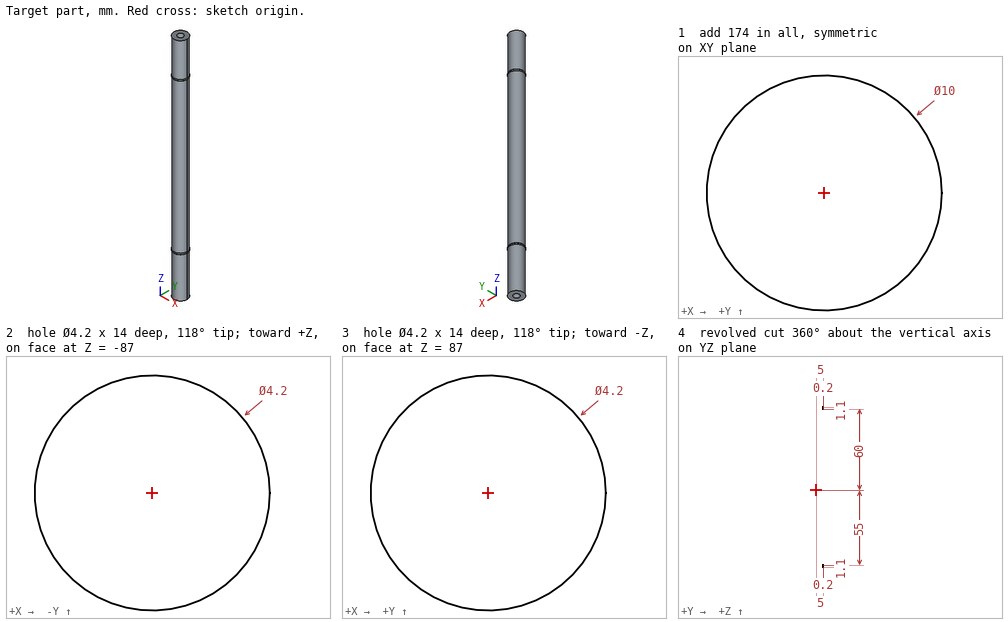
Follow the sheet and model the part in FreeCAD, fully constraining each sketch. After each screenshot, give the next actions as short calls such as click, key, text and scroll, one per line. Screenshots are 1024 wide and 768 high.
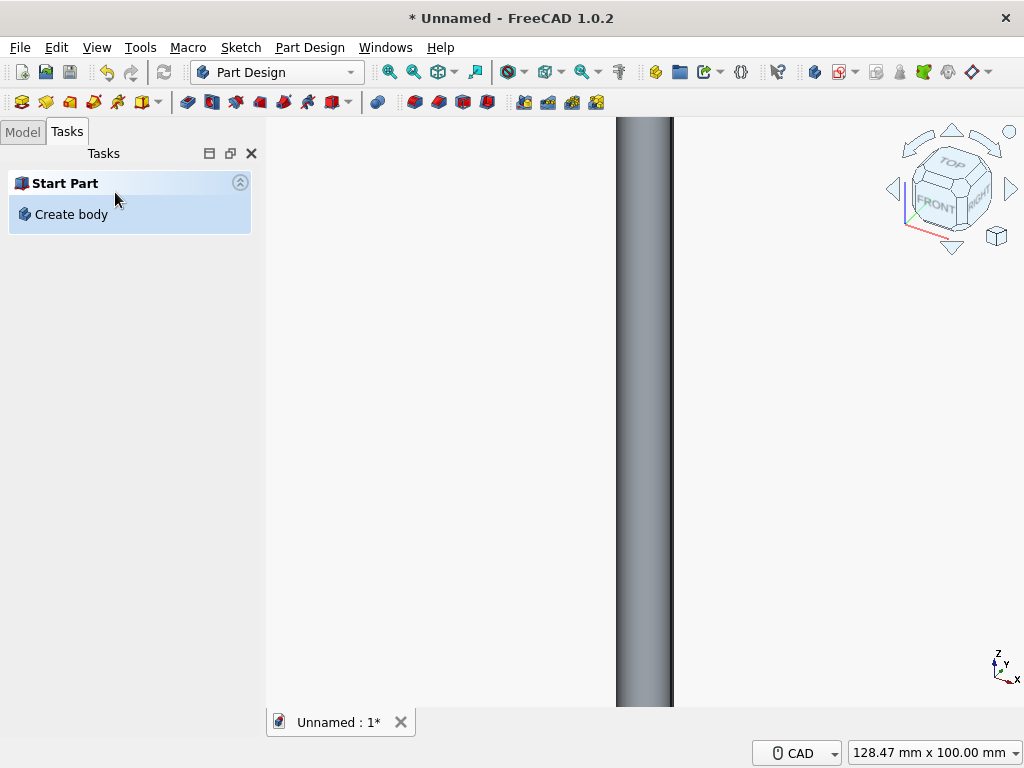
click(390, 72)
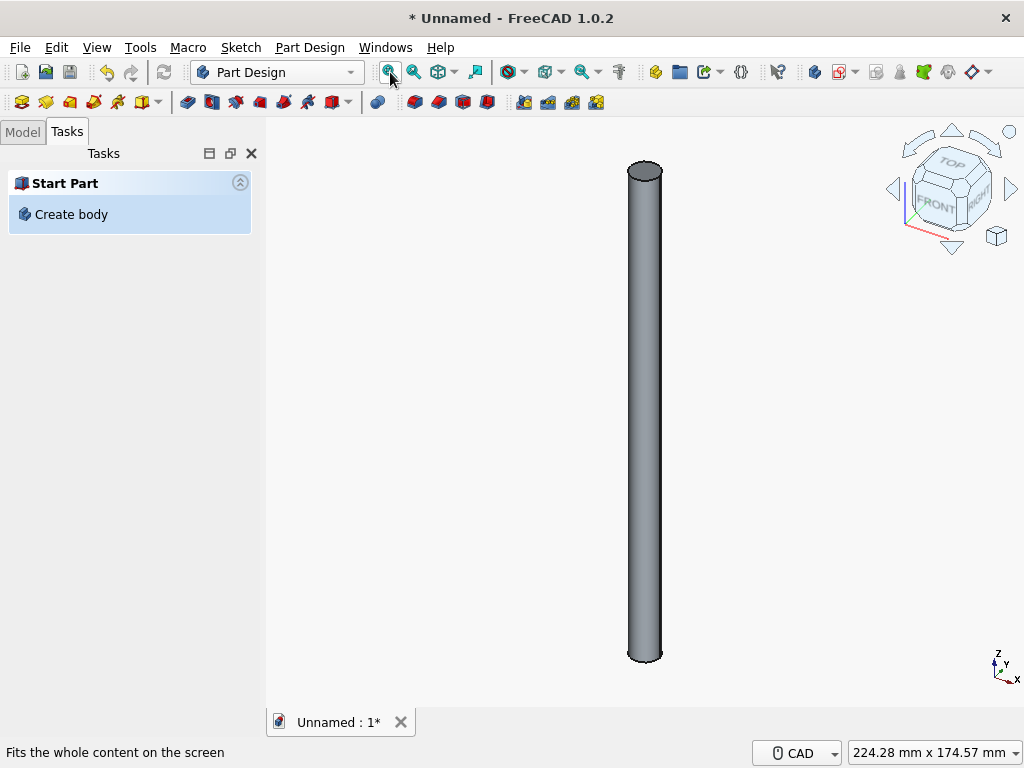
key(5)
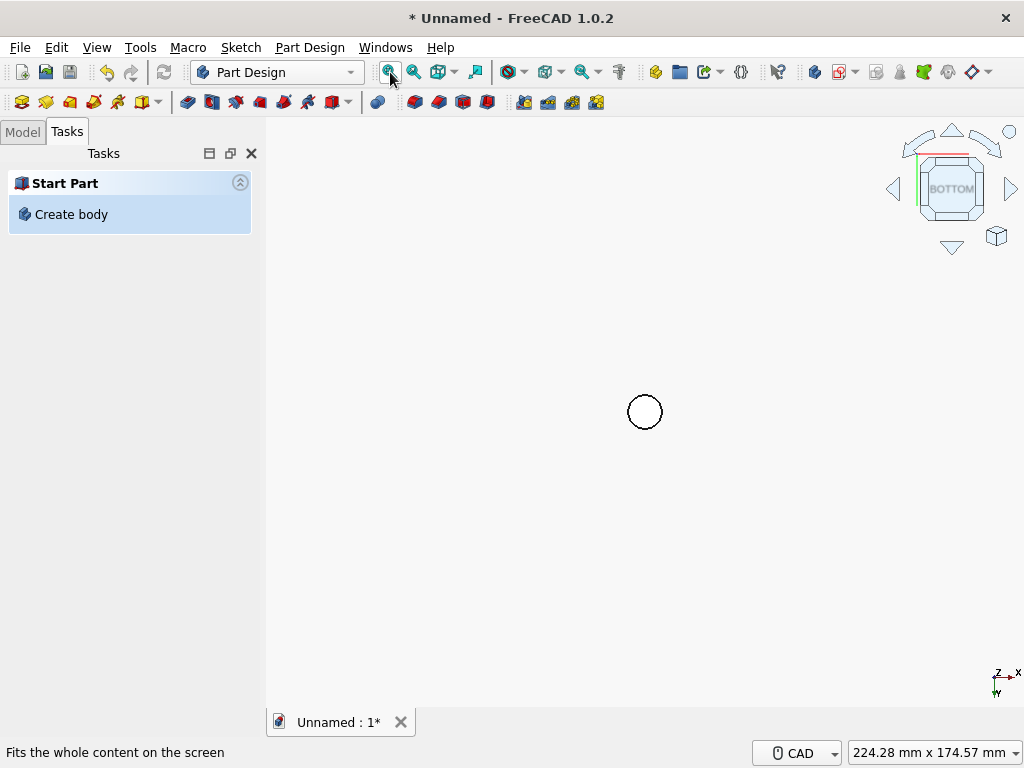
click(390, 72)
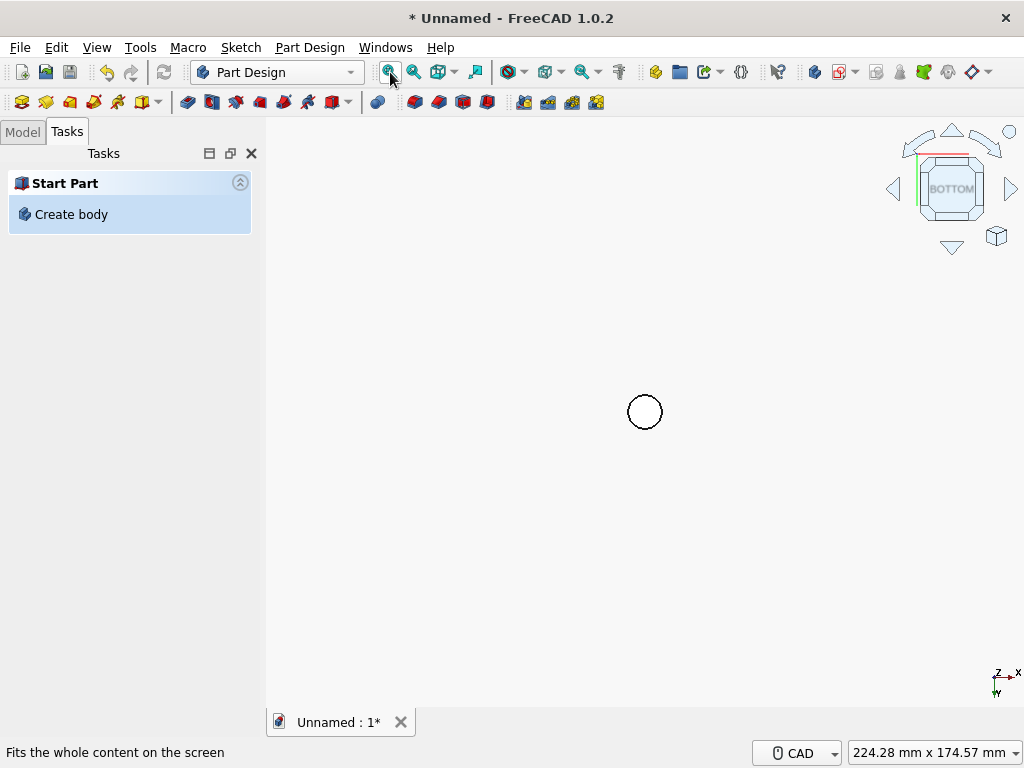
click(645, 411)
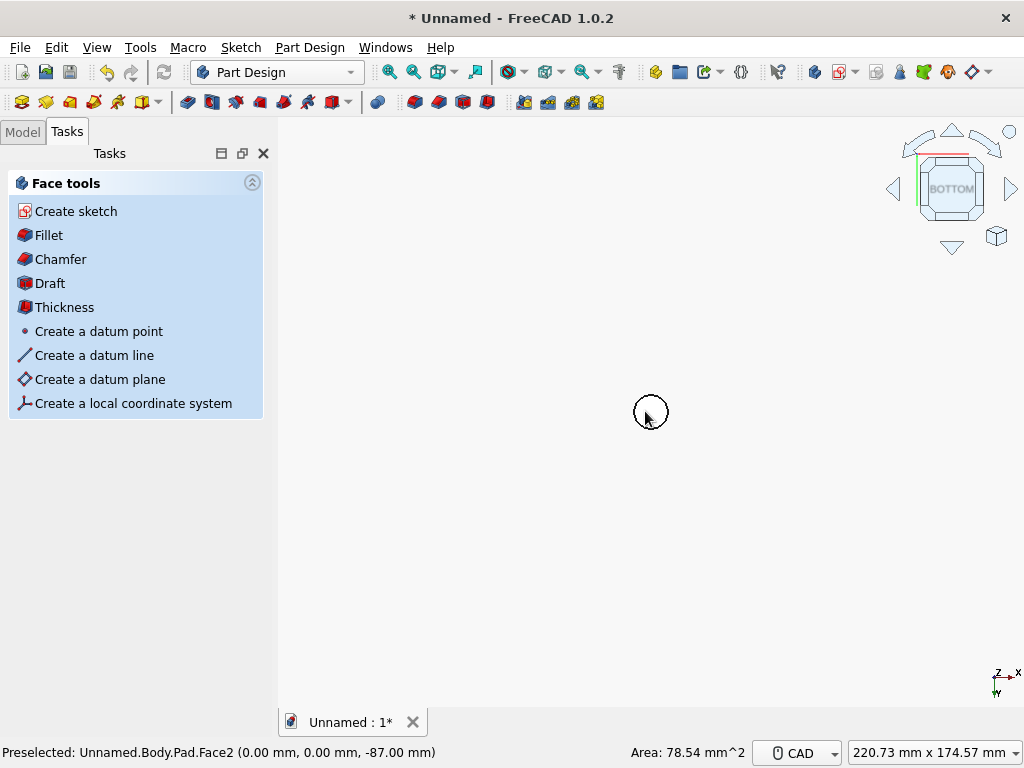
click(840, 72)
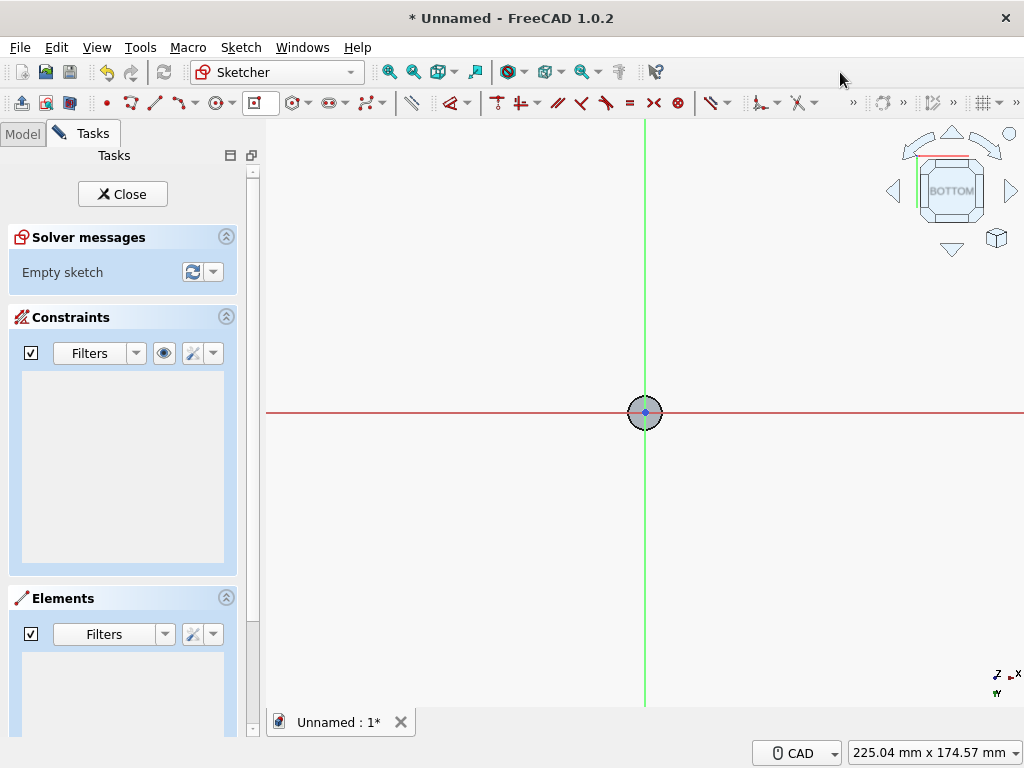
scroll(649, 413, up, 15)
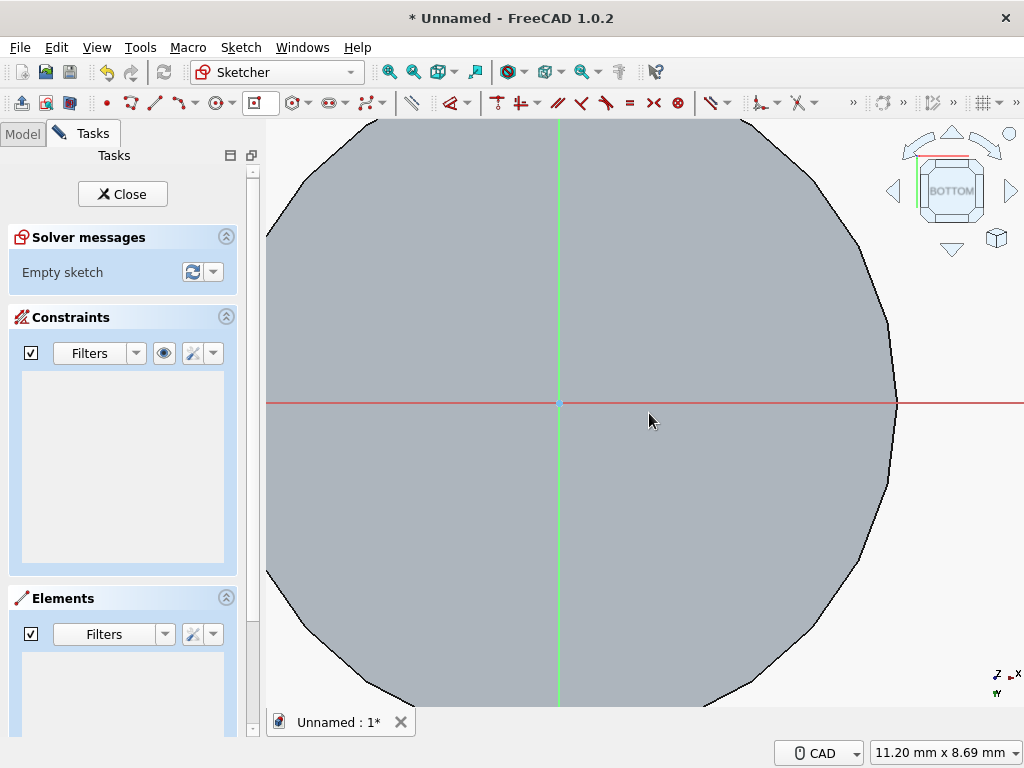
click(216, 104)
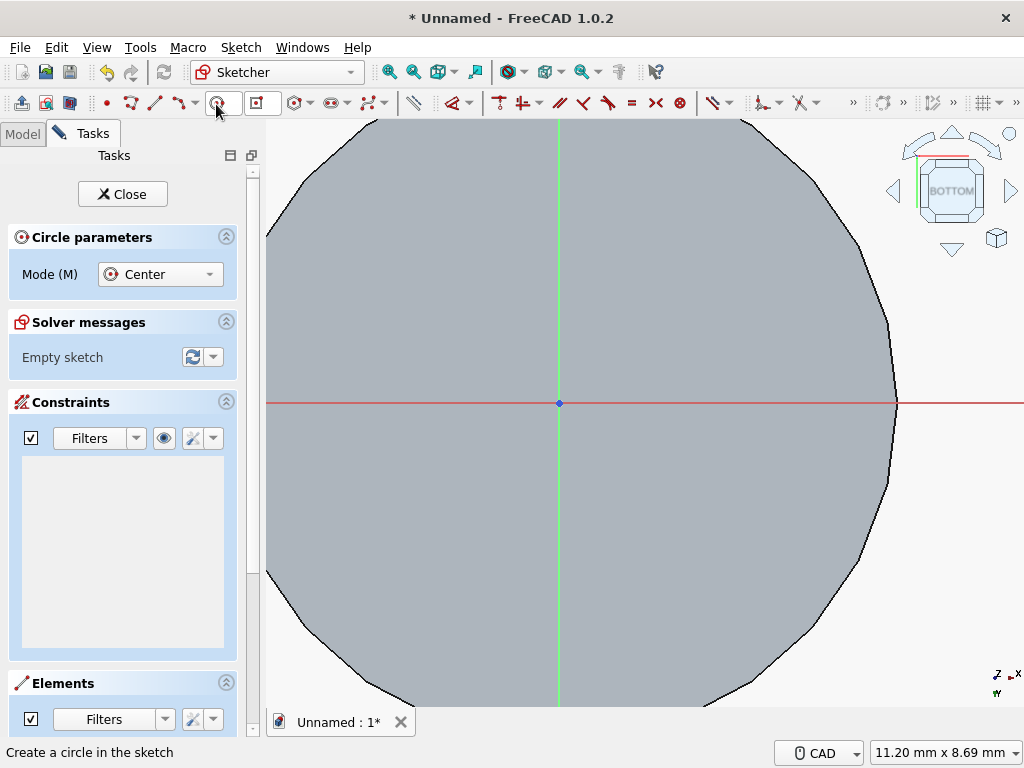
click(559, 403)
move(659, 303)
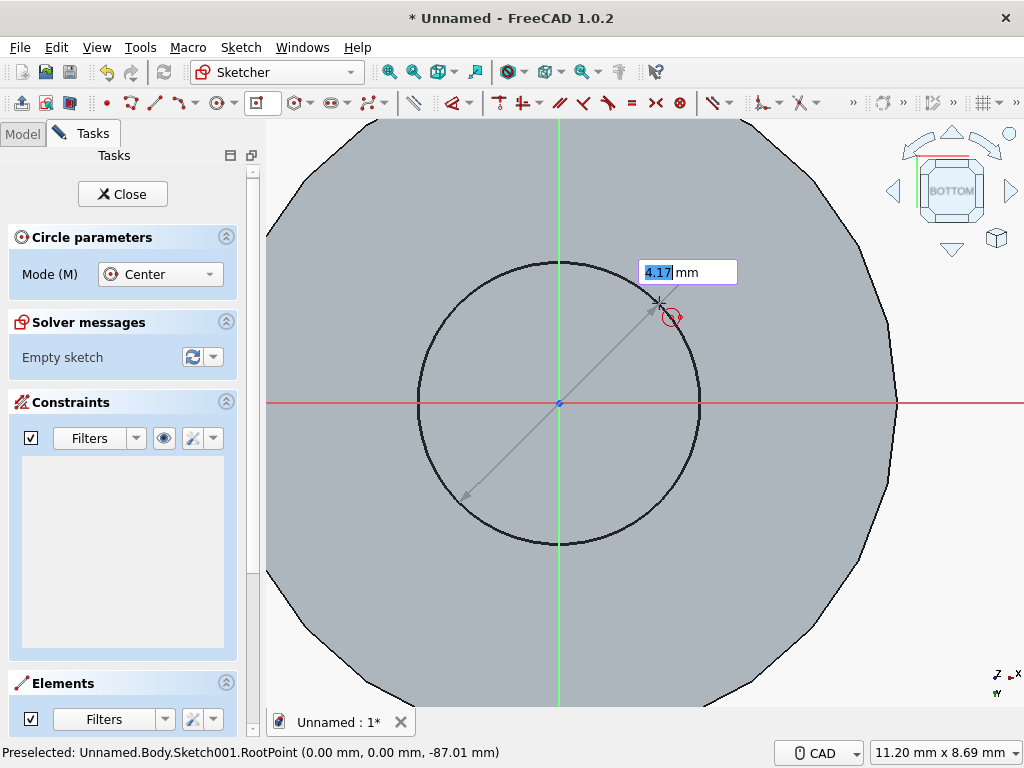
text(4.2)
key(Return)
key(Escape)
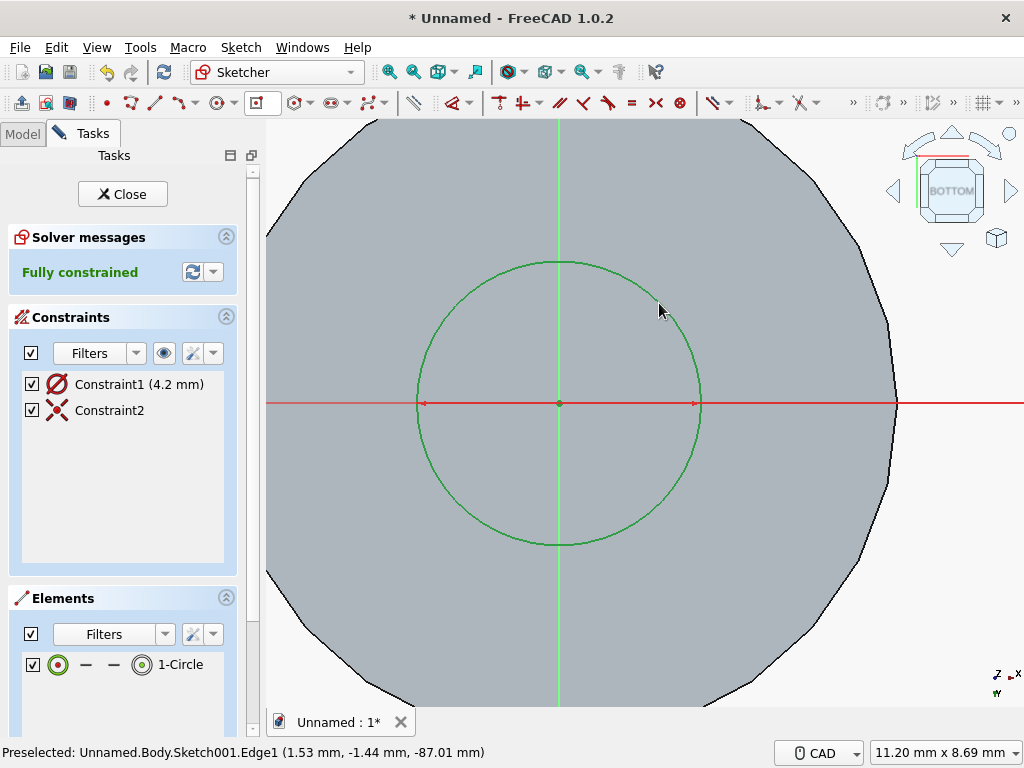
click(123, 194)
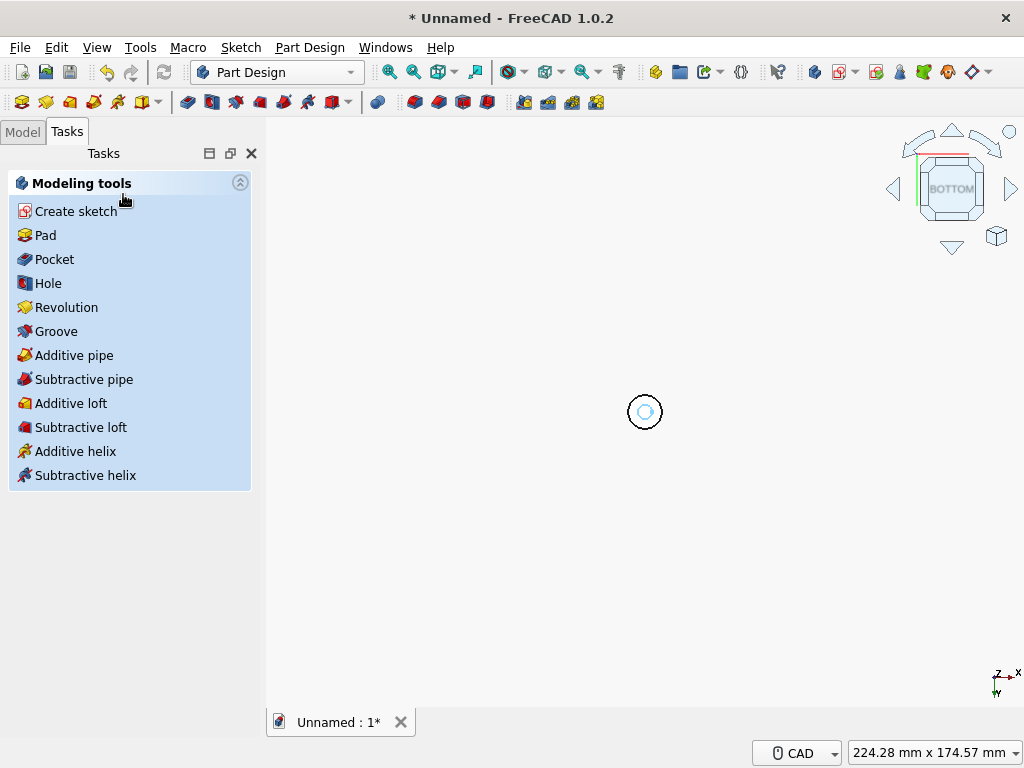
click(212, 102)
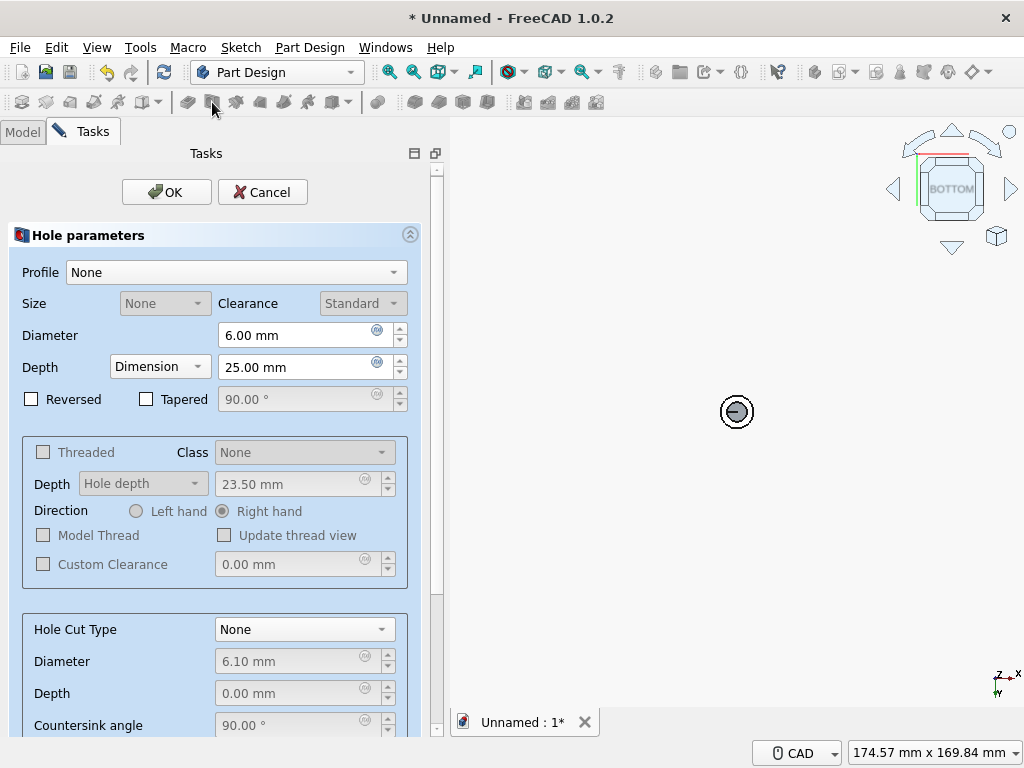
triple_click(305, 335)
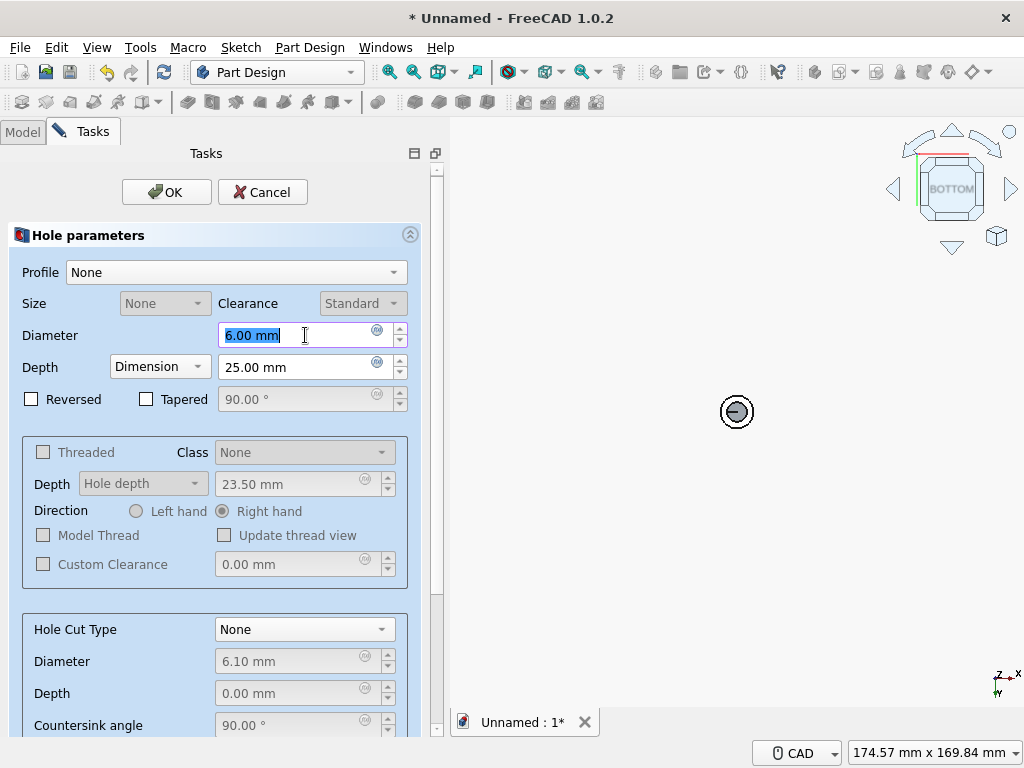
text(4.2)
key(Tab)